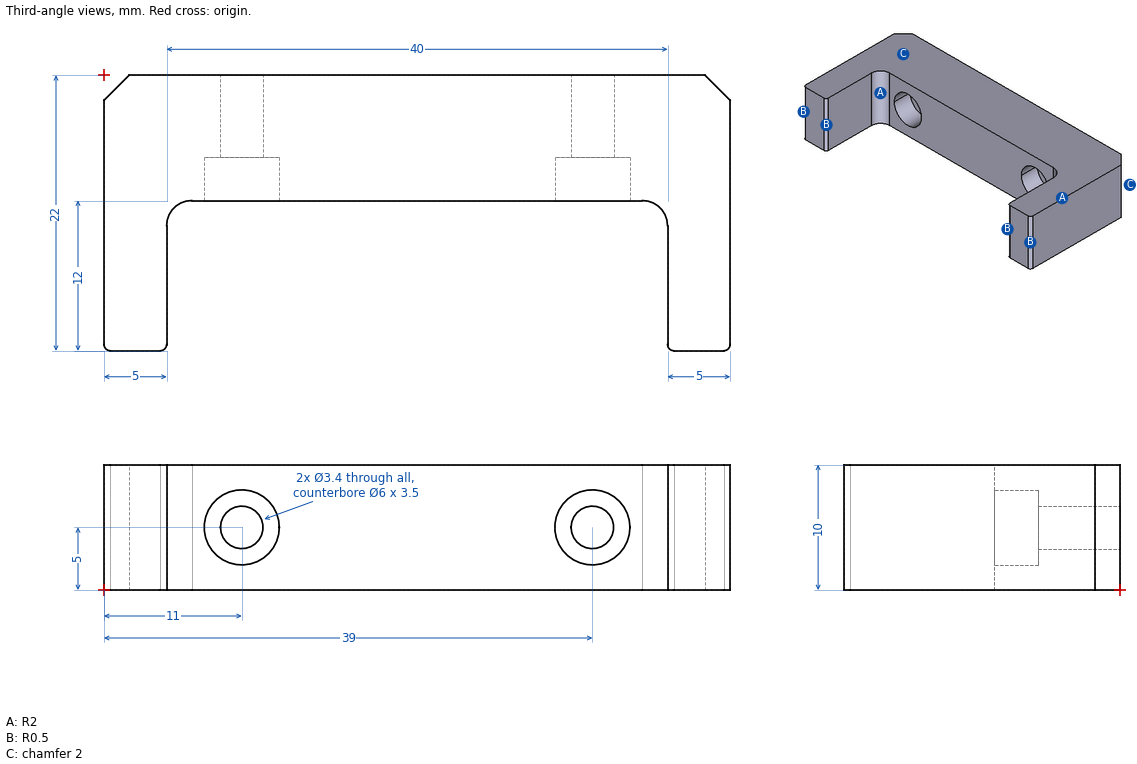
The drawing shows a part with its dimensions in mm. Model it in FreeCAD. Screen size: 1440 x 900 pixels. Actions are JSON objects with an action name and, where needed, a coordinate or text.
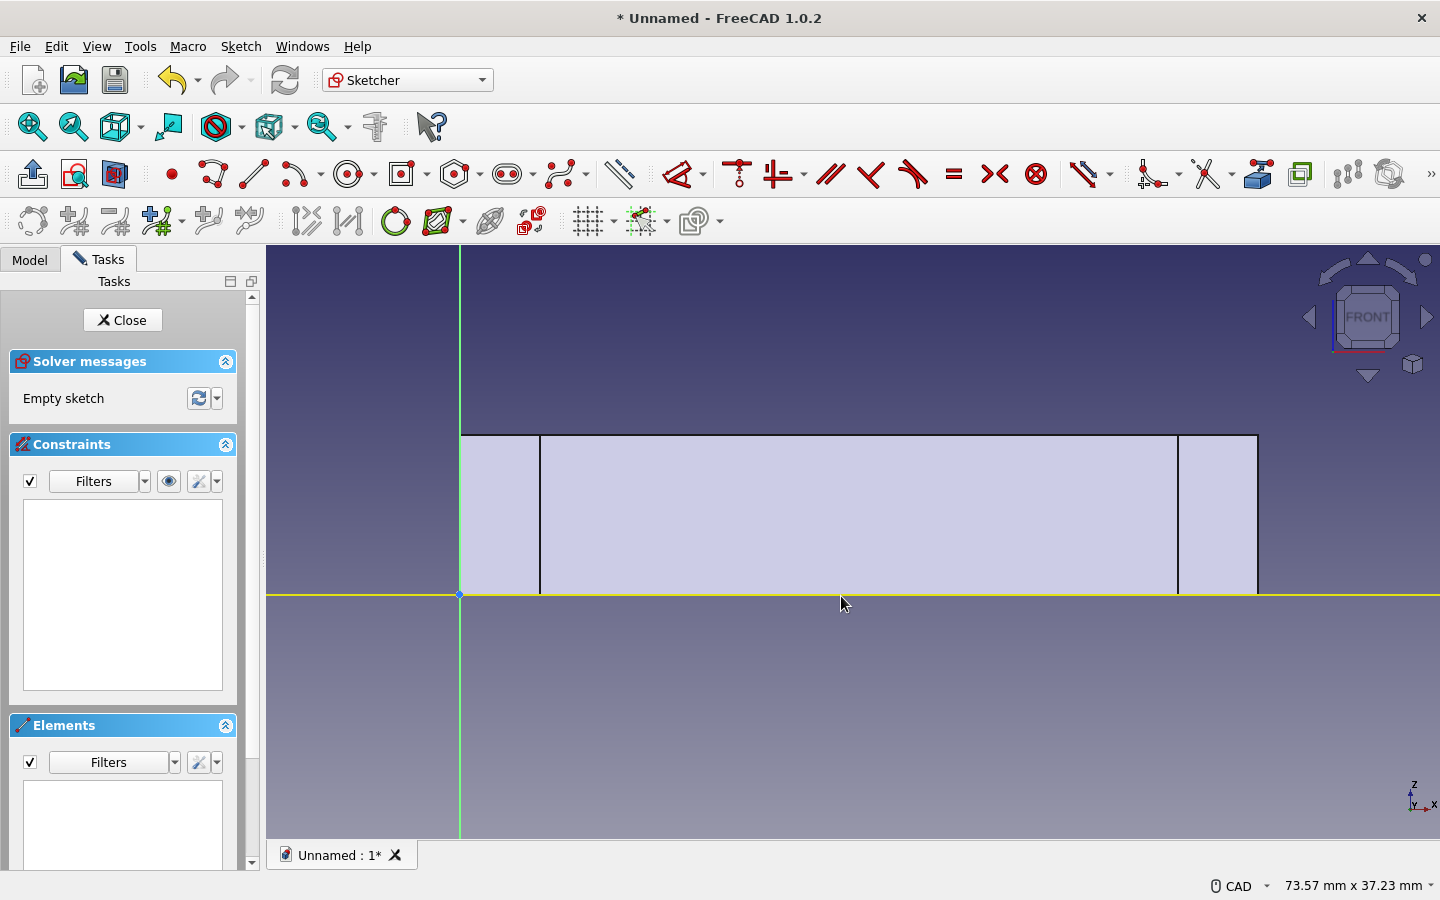
{"action": "left_click", "coordinate": [348, 174]}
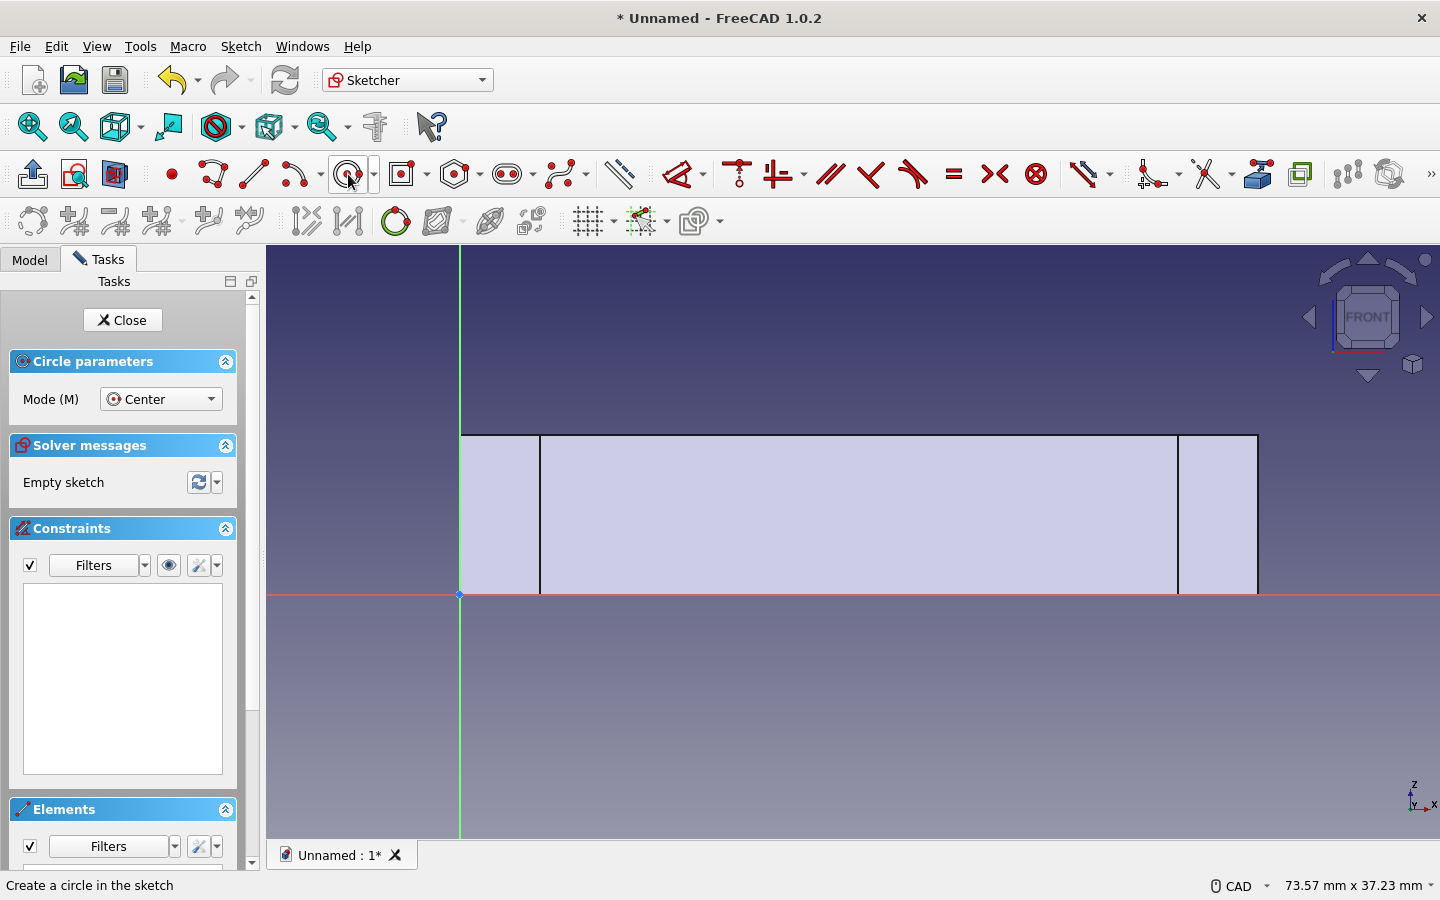
{"action": "left_click", "coordinate": [635, 515]}
{"action": "left_click", "coordinate": [654, 496]}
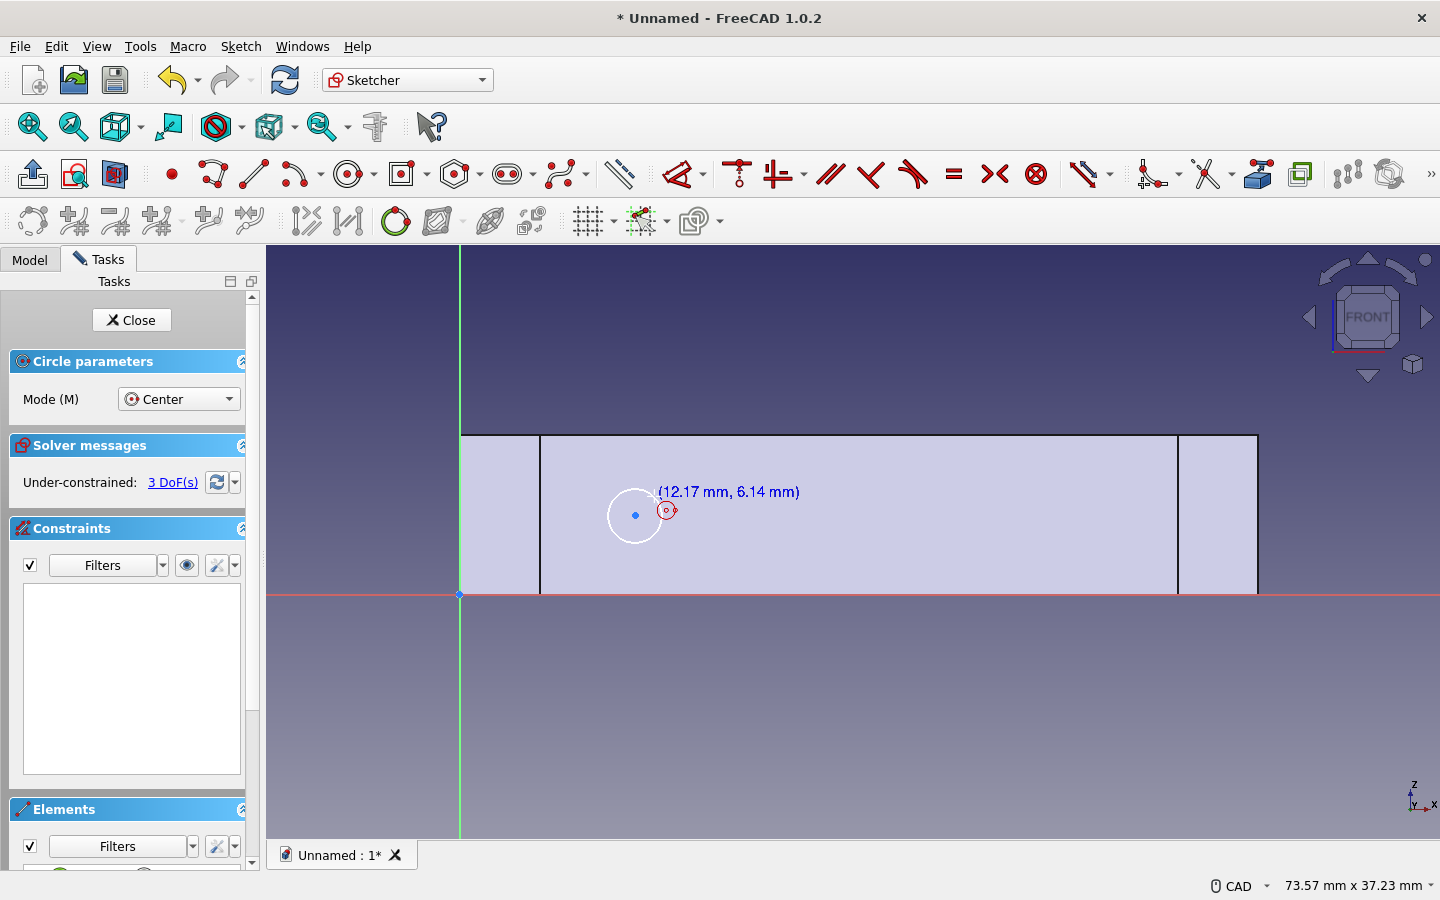
{"action": "left_click", "coordinate": [1082, 515]}
{"action": "left_click", "coordinate": [1101, 496]}
{"action": "key", "text": "Escape"}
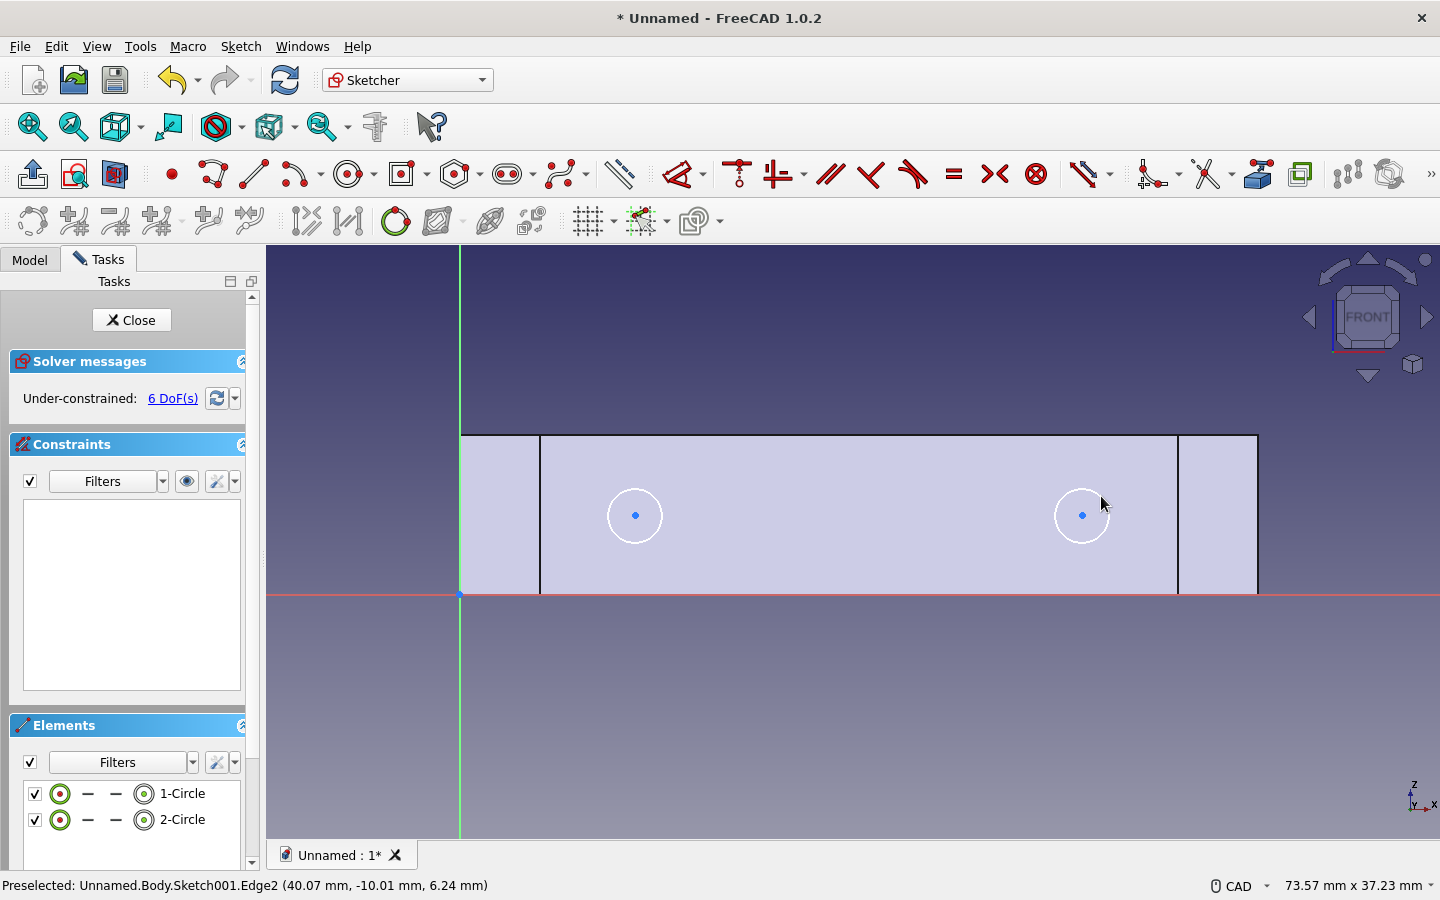
{"action": "left_click", "coordinate": [654, 497]}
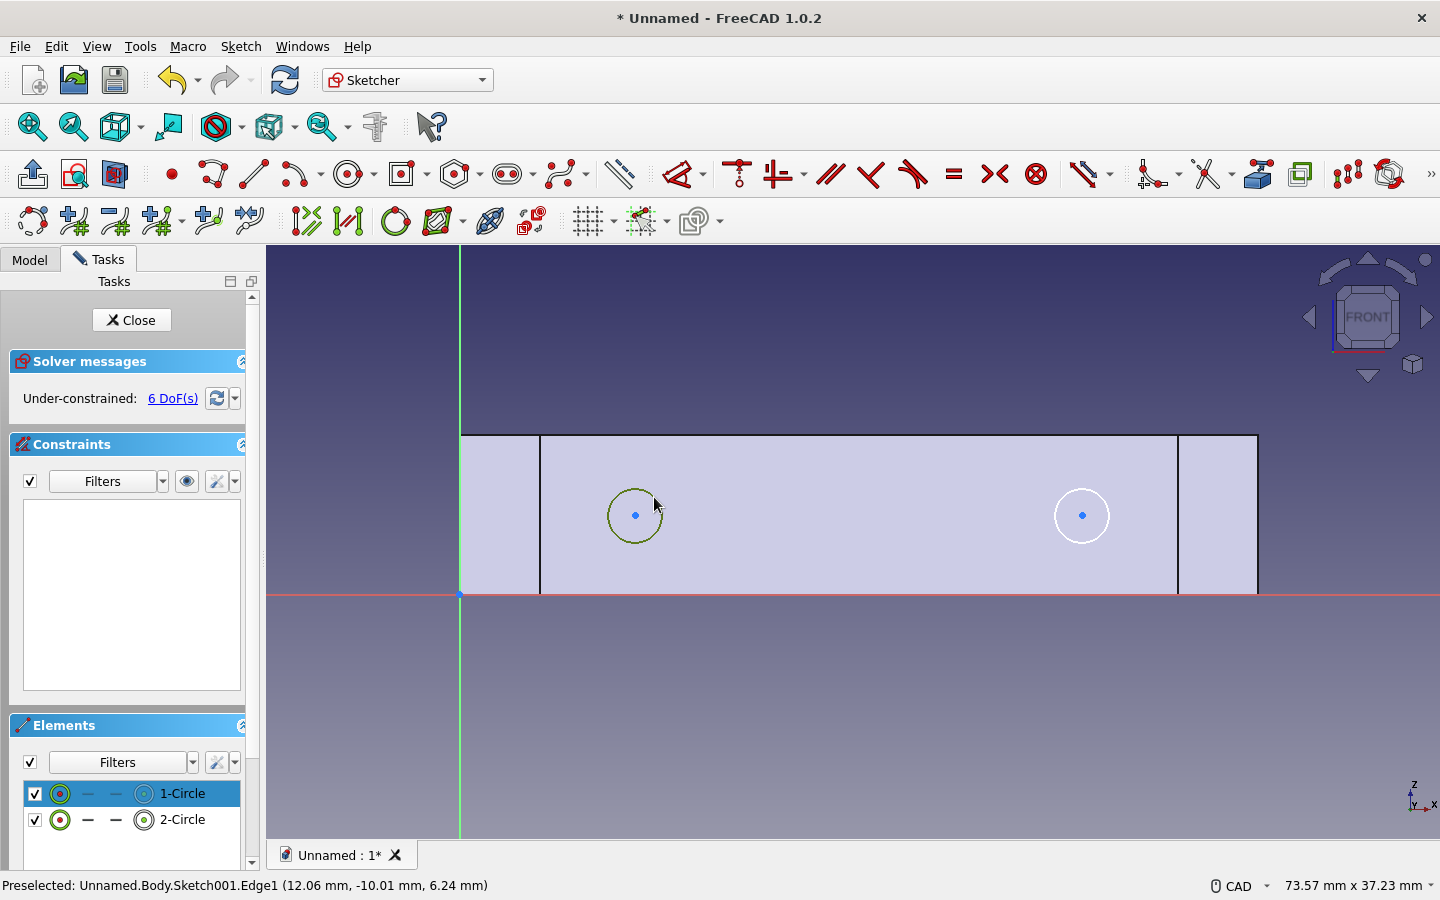
{"action": "left_click", "coordinate": [1101, 497]}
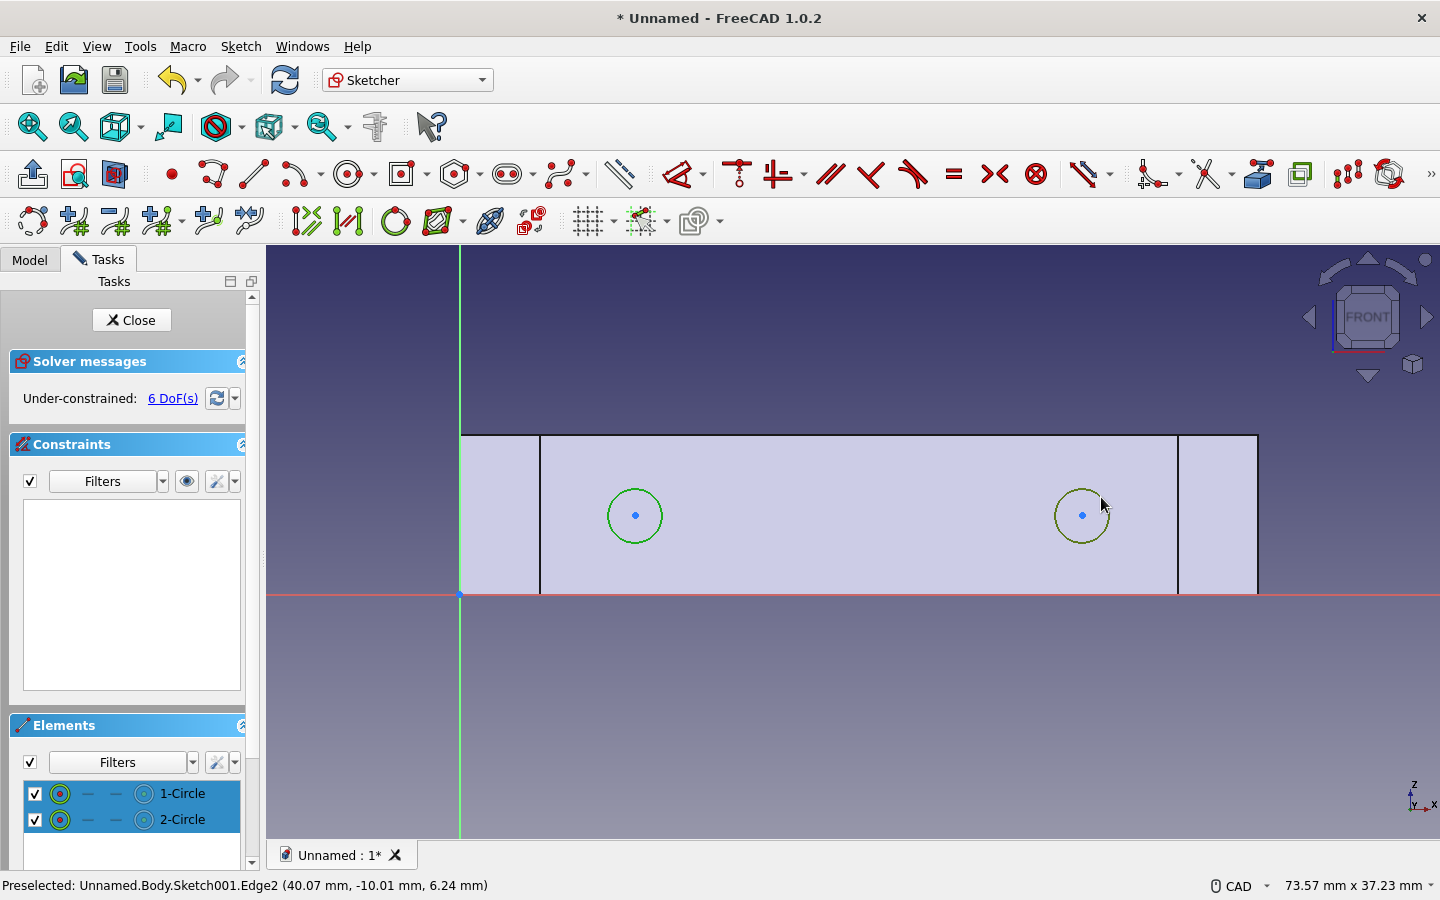
{"action": "left_click", "coordinate": [954, 174]}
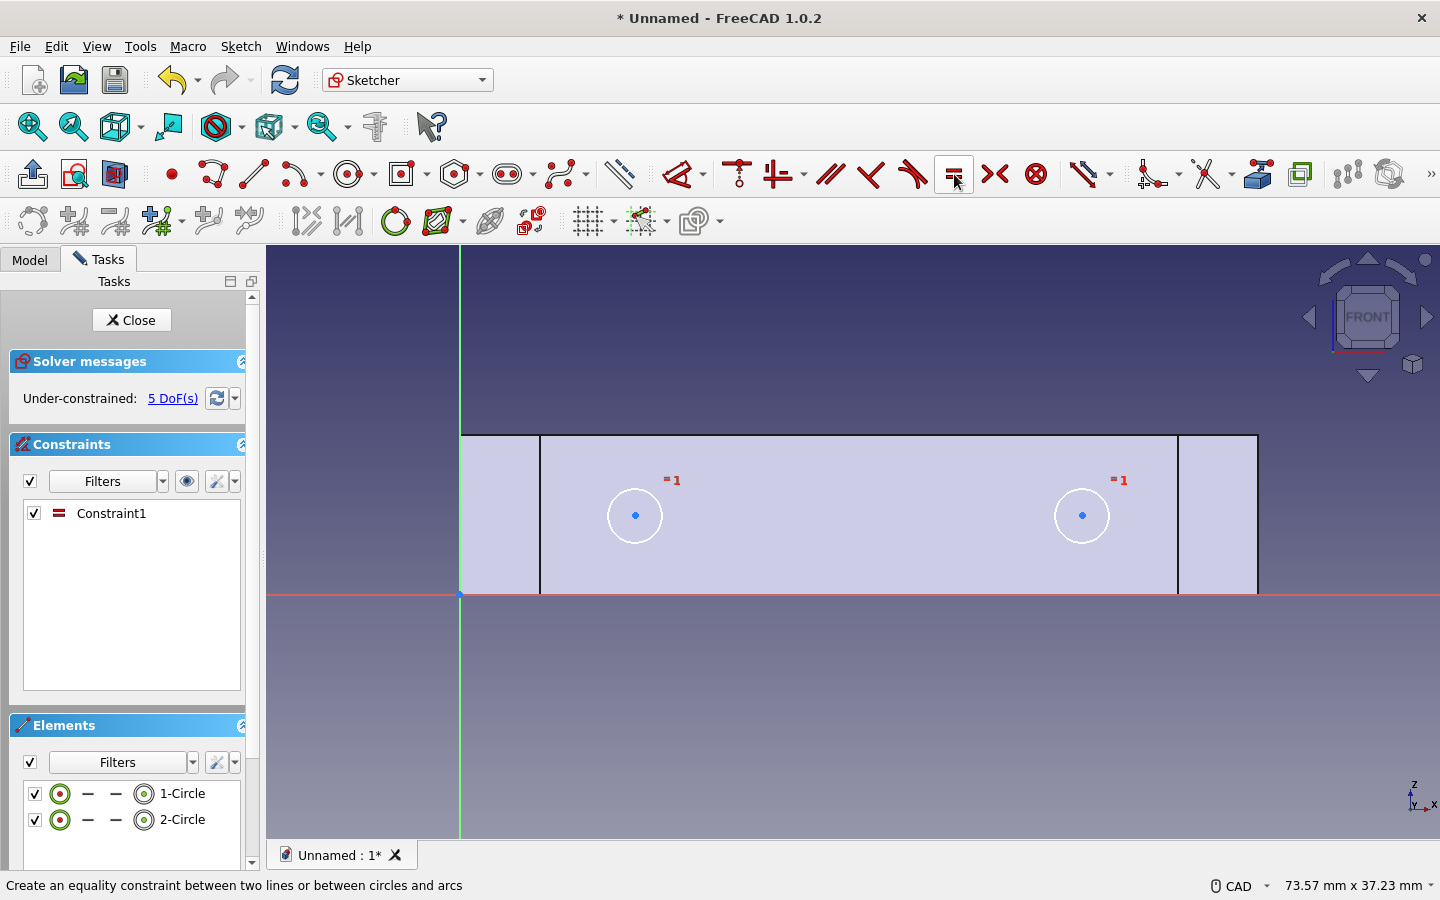
{"action": "left_click", "coordinate": [635, 516]}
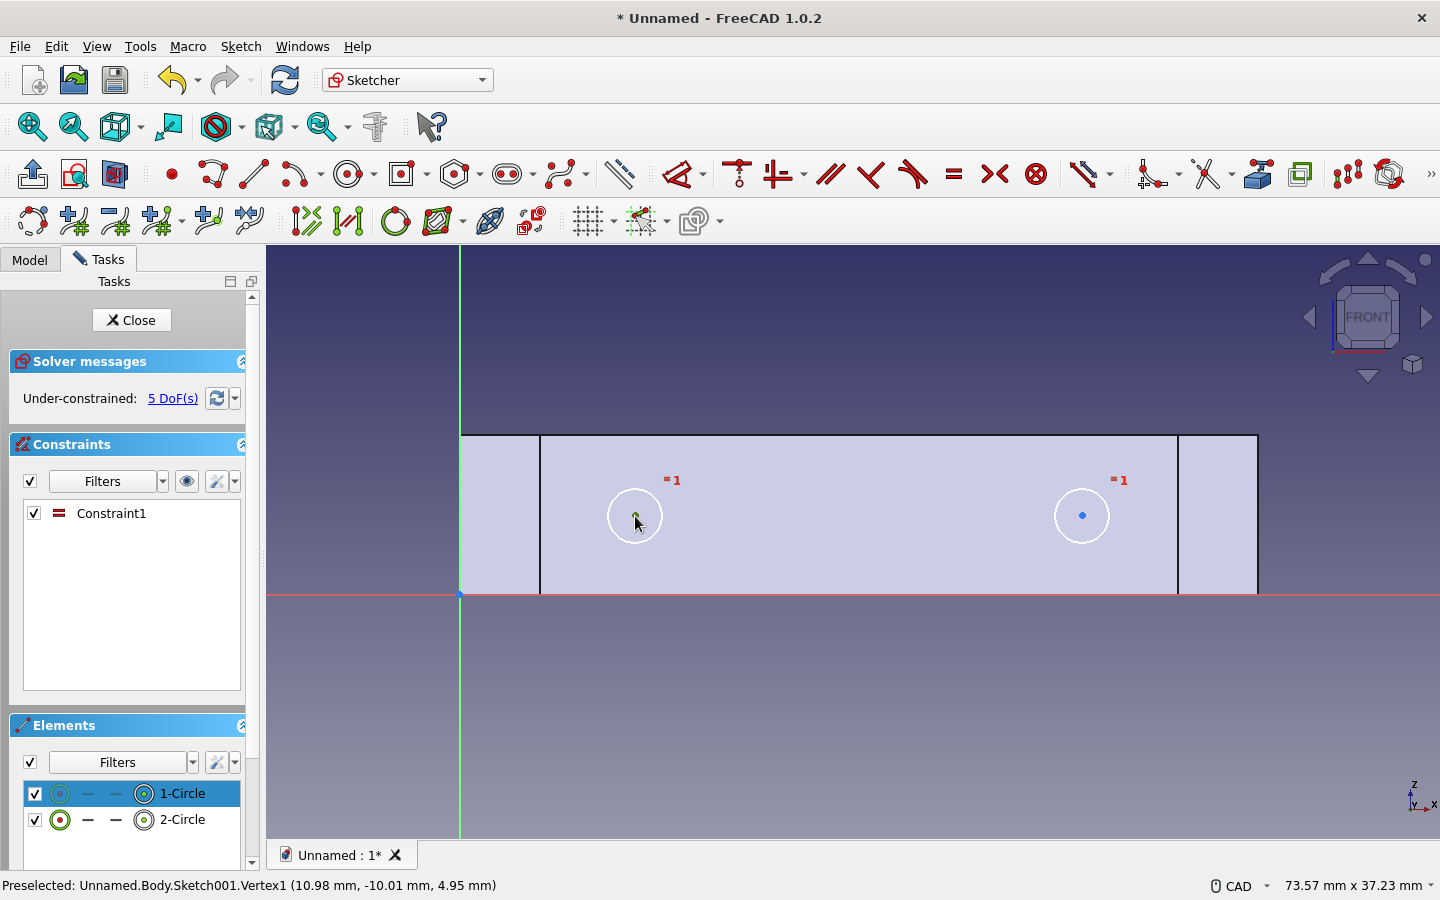
{"action": "left_click", "coordinate": [1082, 516]}